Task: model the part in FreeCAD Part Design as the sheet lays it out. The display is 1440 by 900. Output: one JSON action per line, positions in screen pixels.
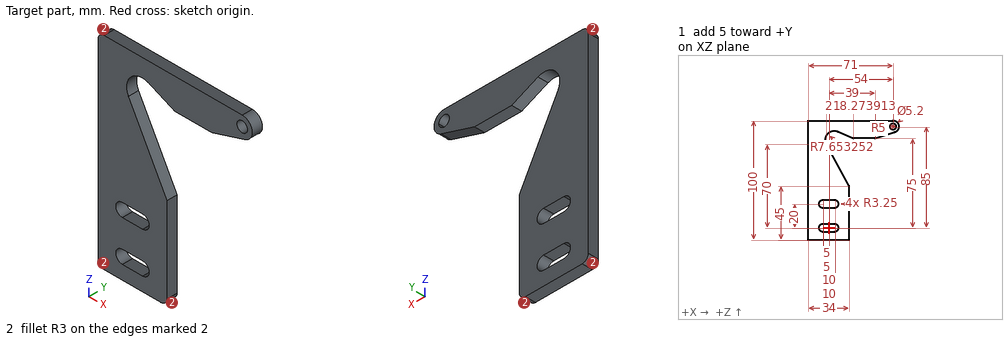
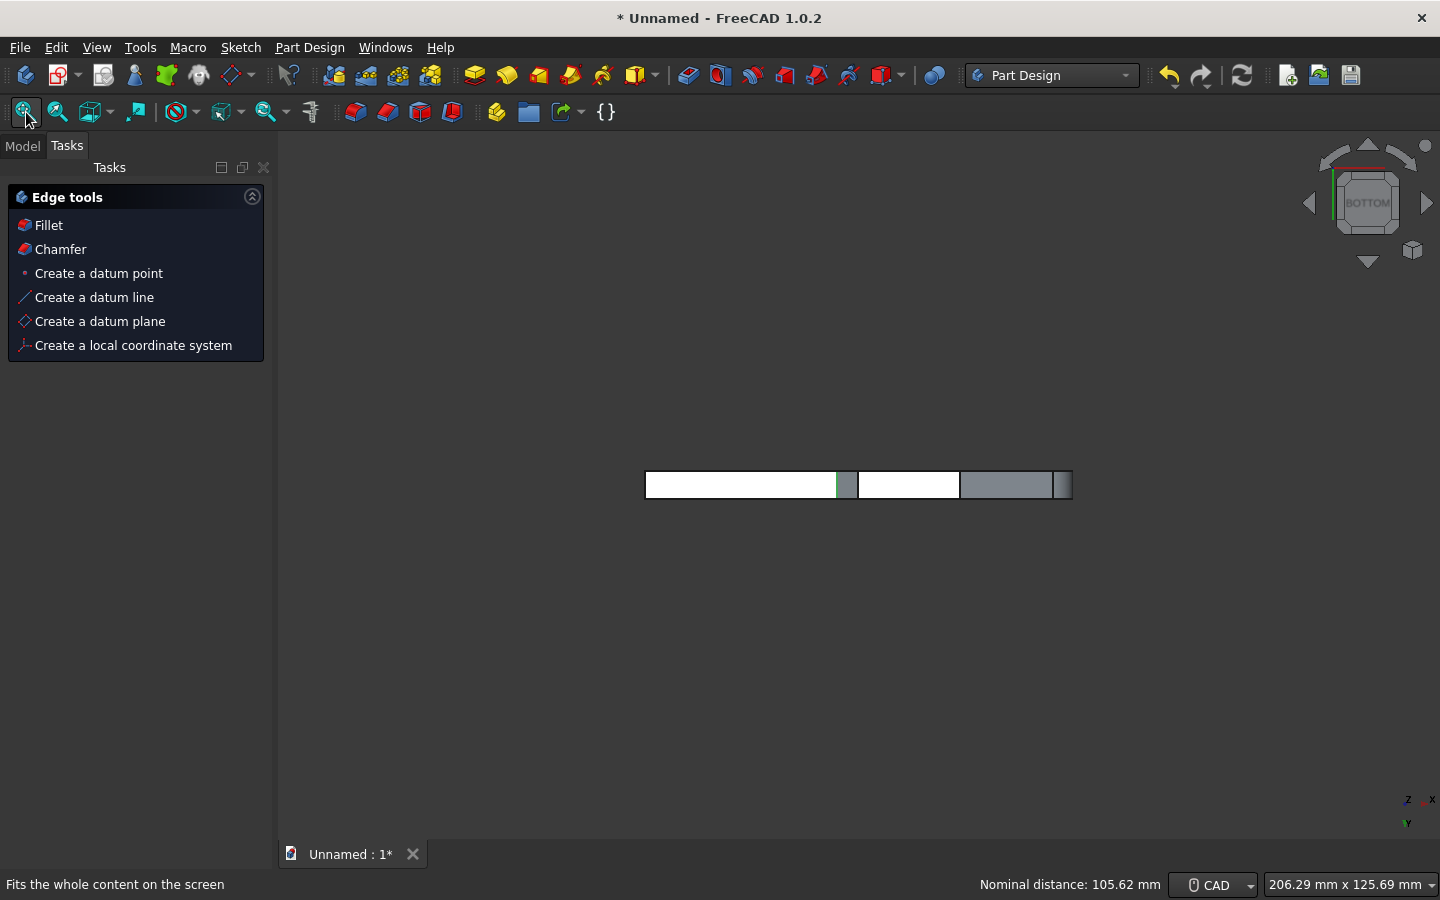
{"action": "left_click", "coordinate": [645, 484], "text": "ctrl"}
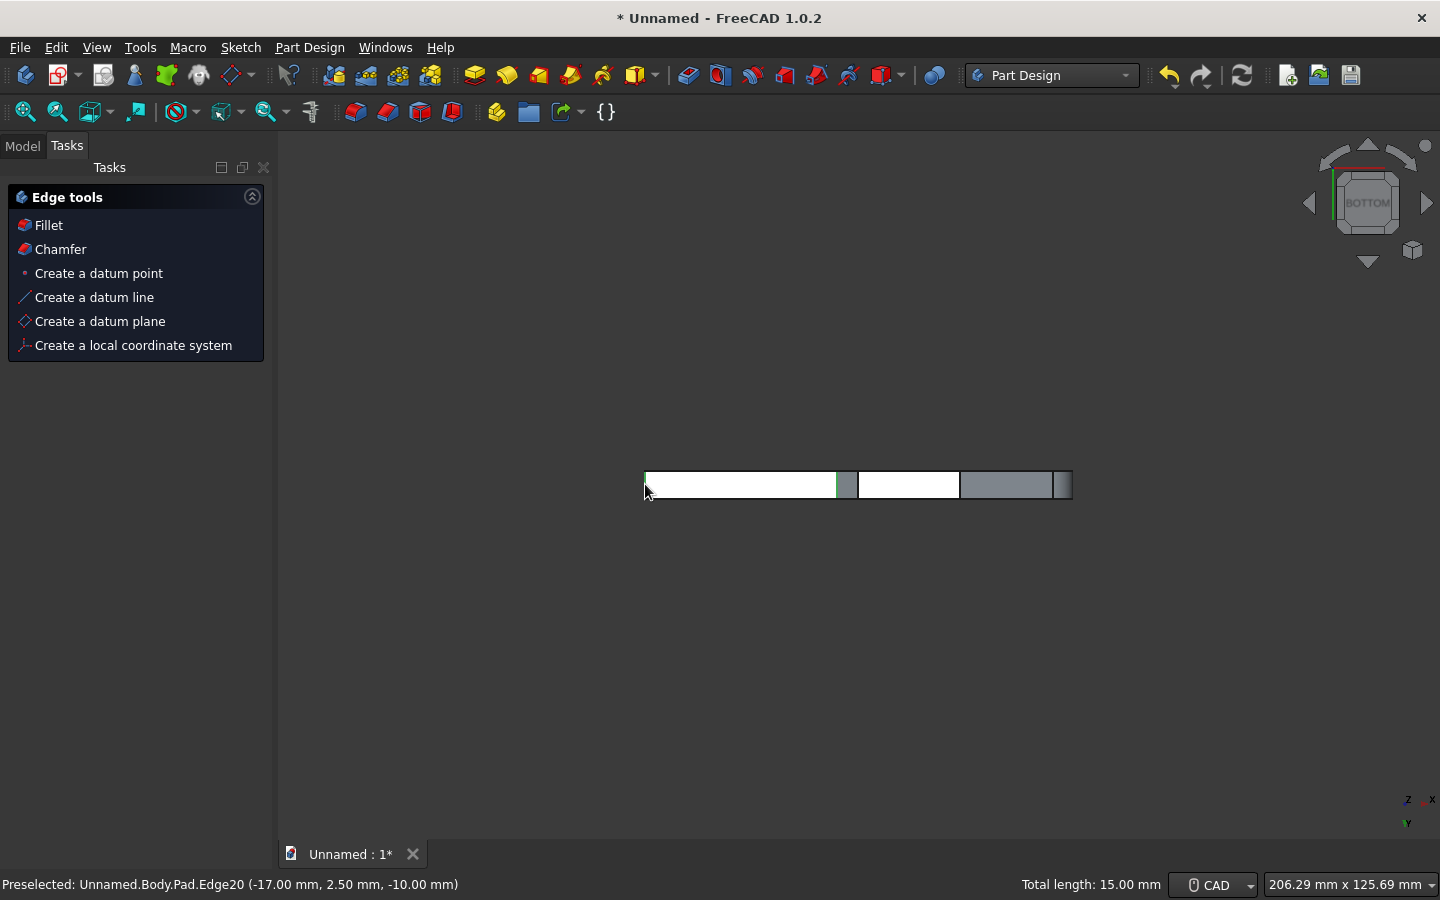
{"action": "left_click", "coordinate": [356, 112]}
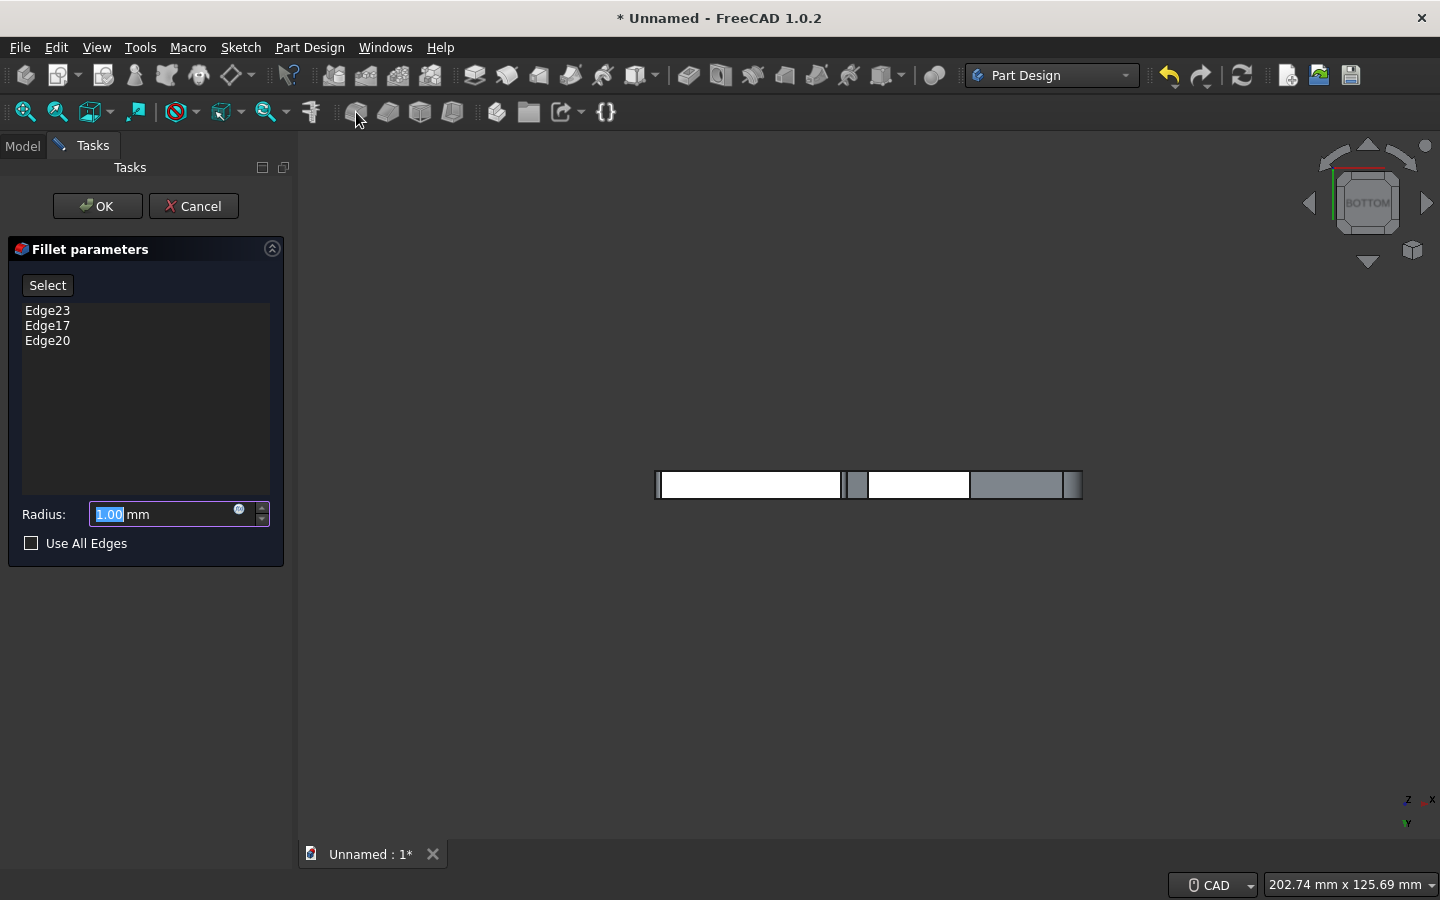
{"action": "type", "text": "3"}
{"action": "key", "text": "Tab"}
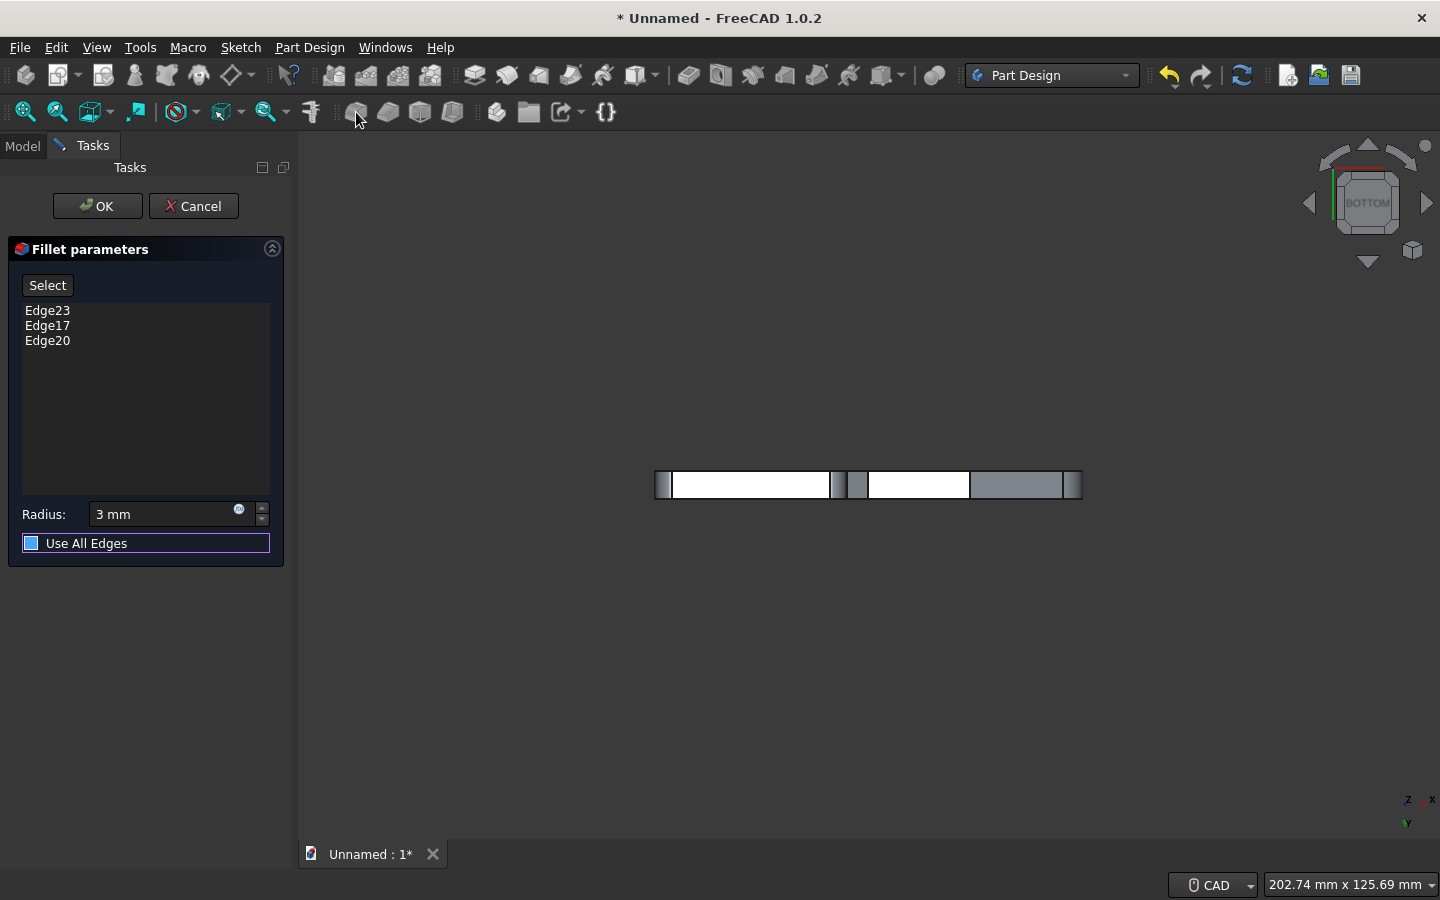
{"action": "left_click", "coordinate": [98, 206]}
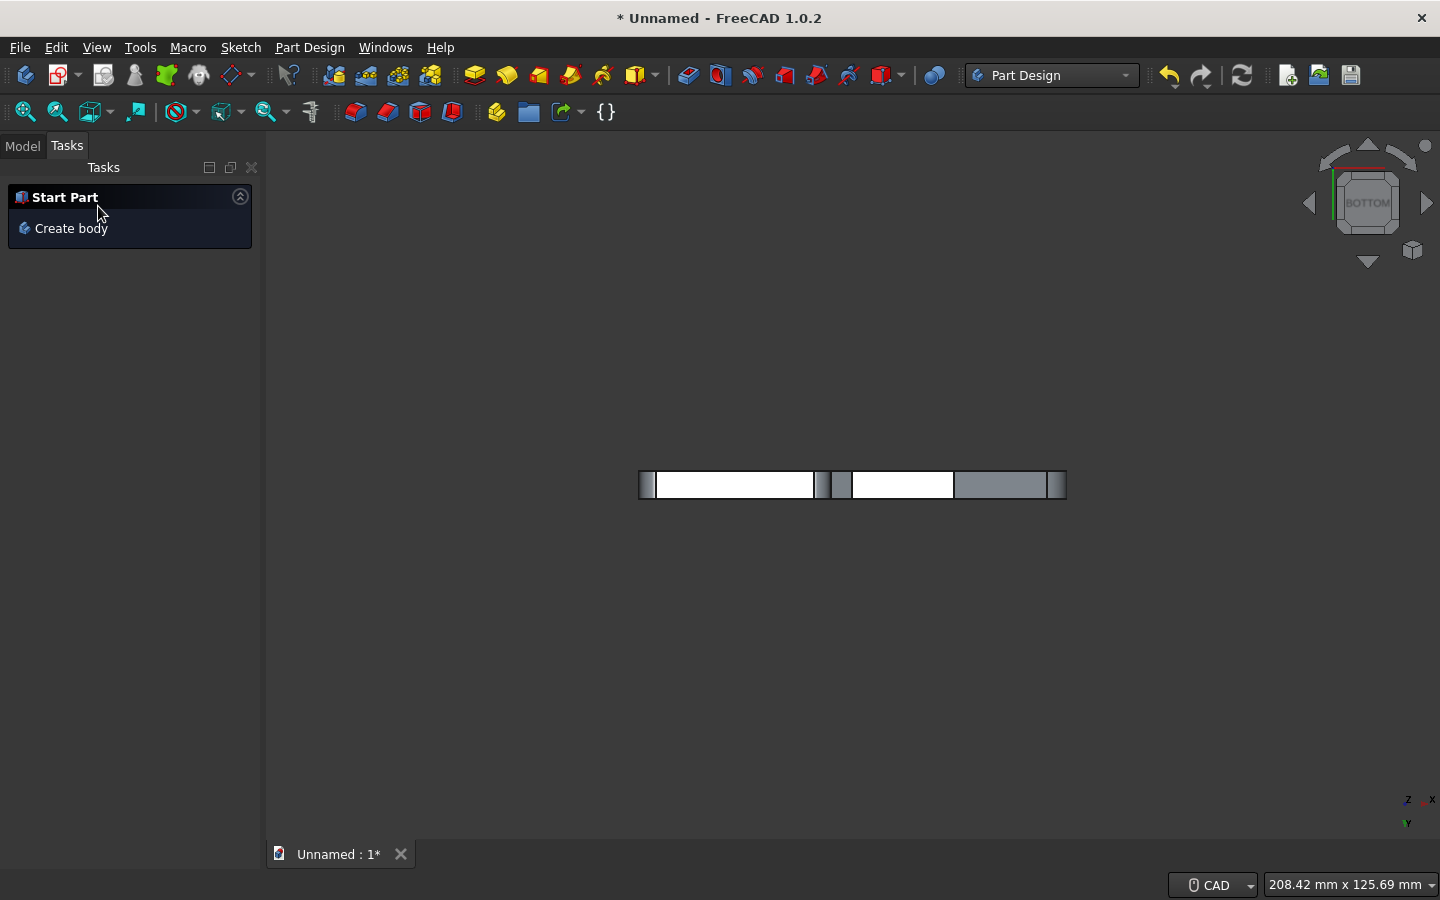
{"action": "key", "text": "0"}